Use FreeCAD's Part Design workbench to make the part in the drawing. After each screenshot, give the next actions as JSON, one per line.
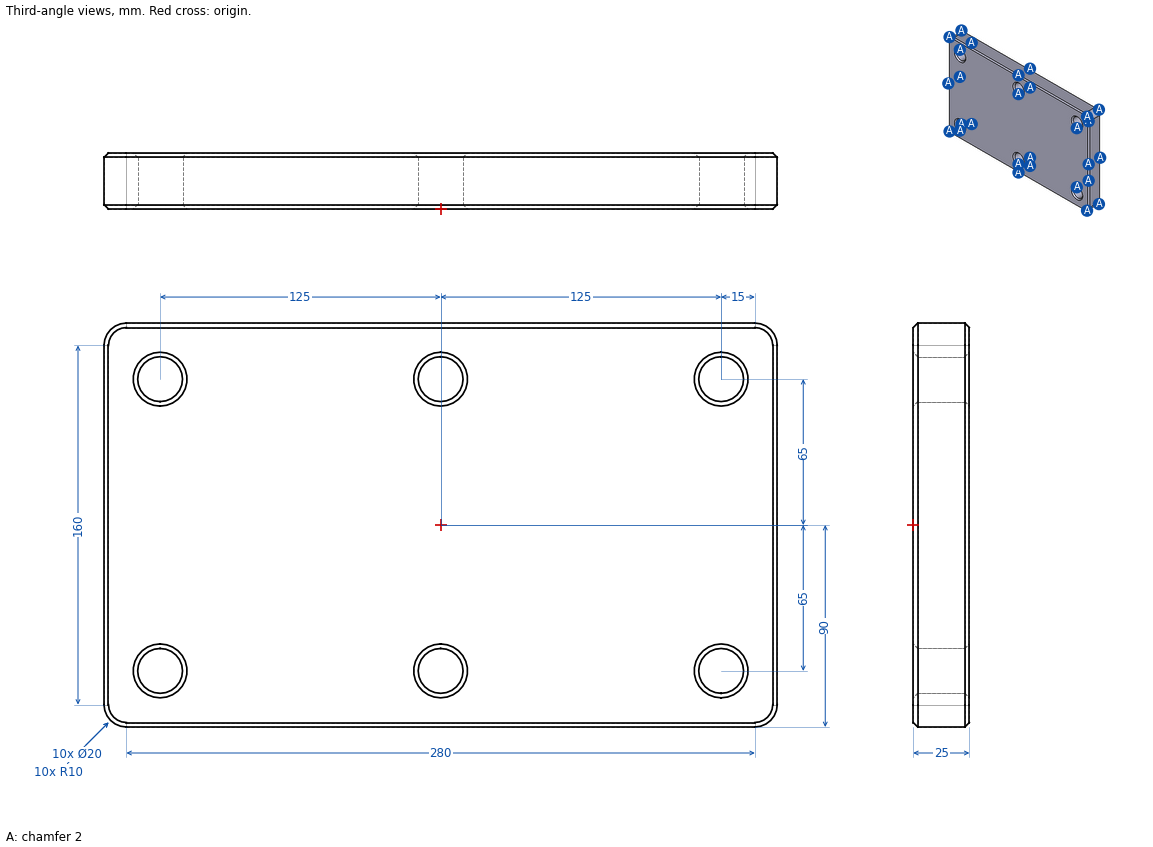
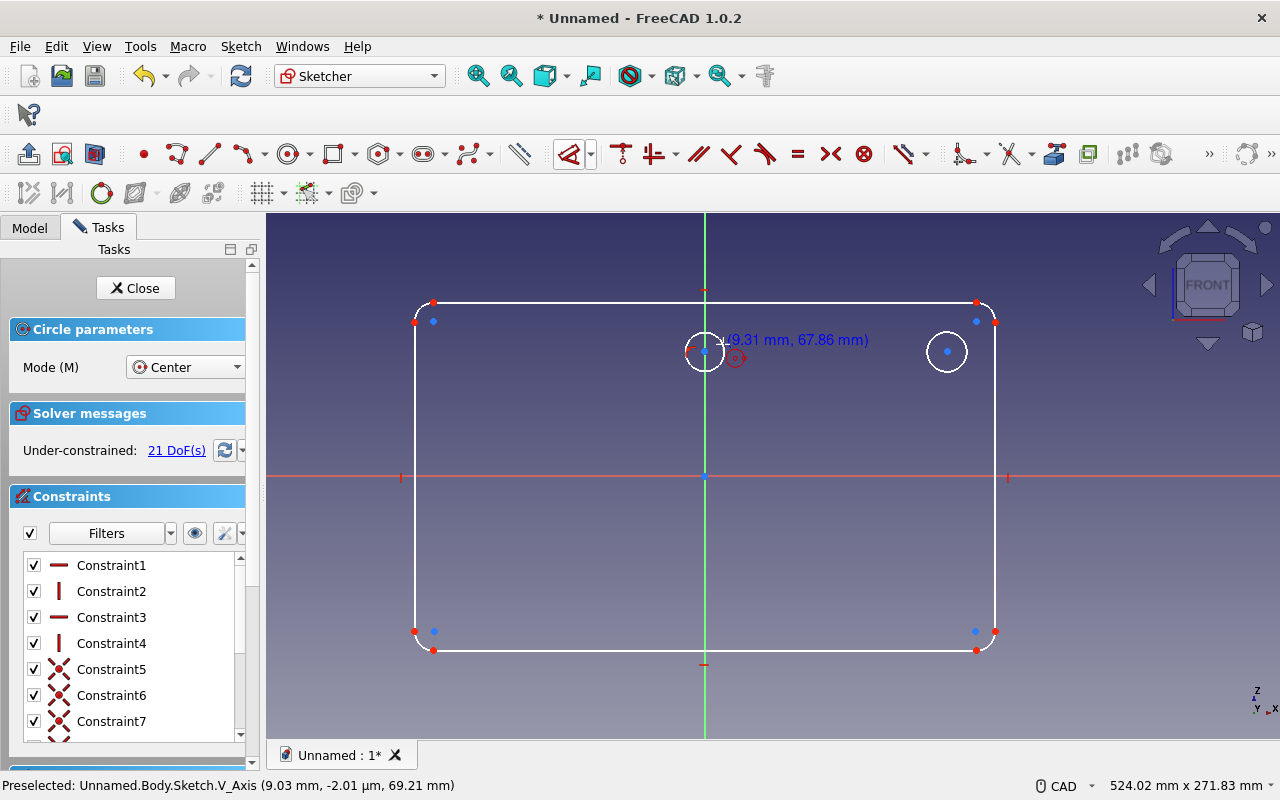
{"action": "left_click", "coordinate": [463, 351]}
{"action": "left_click", "coordinate": [477, 337]}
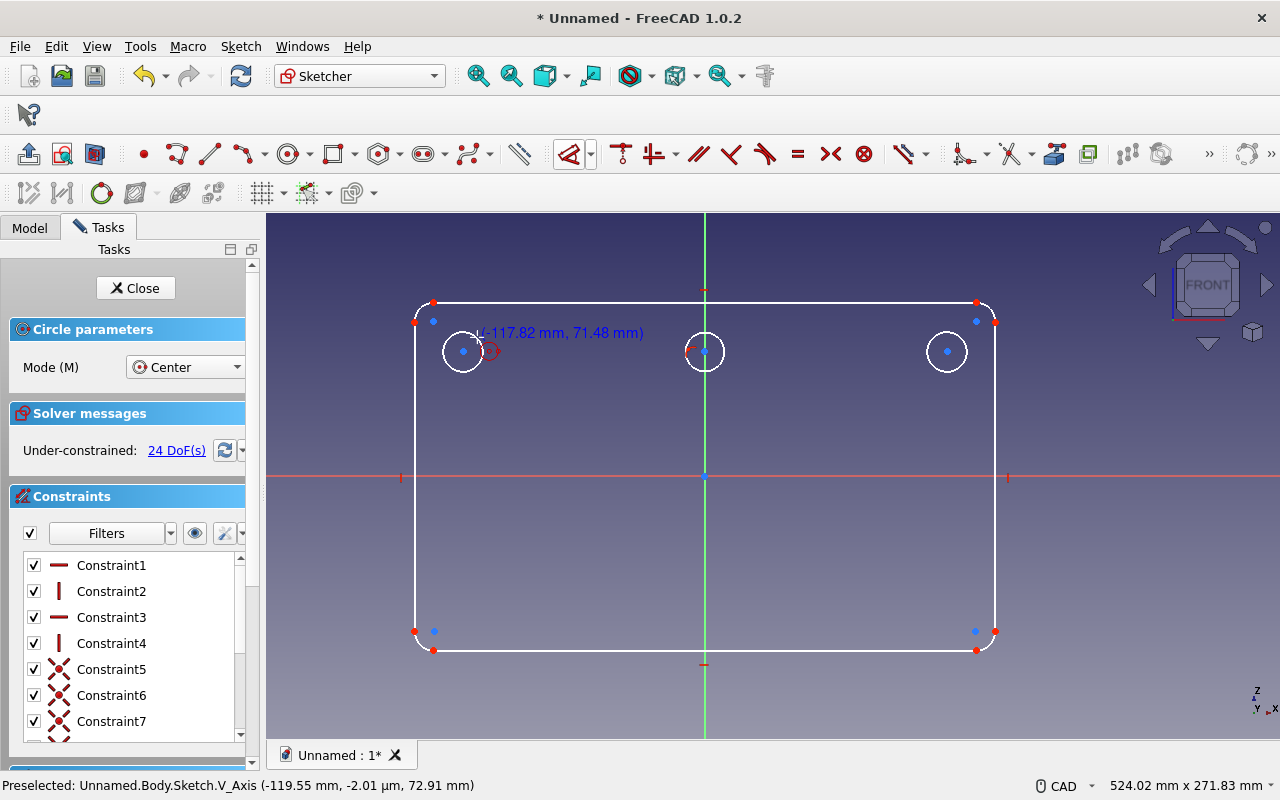
{"action": "left_click", "coordinate": [947, 602]}
{"action": "left_click", "coordinate": [961, 588]}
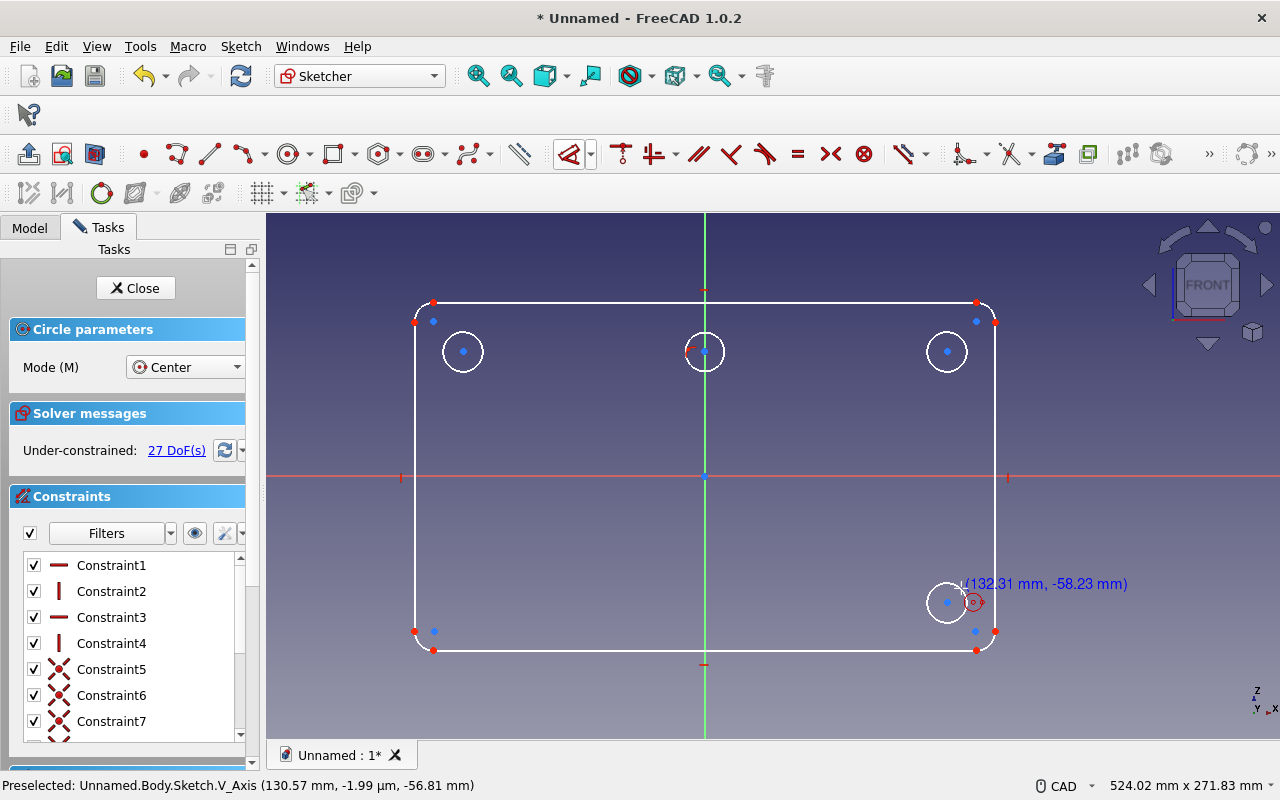
{"action": "left_click", "coordinate": [705, 602]}
{"action": "left_click", "coordinate": [723, 595]}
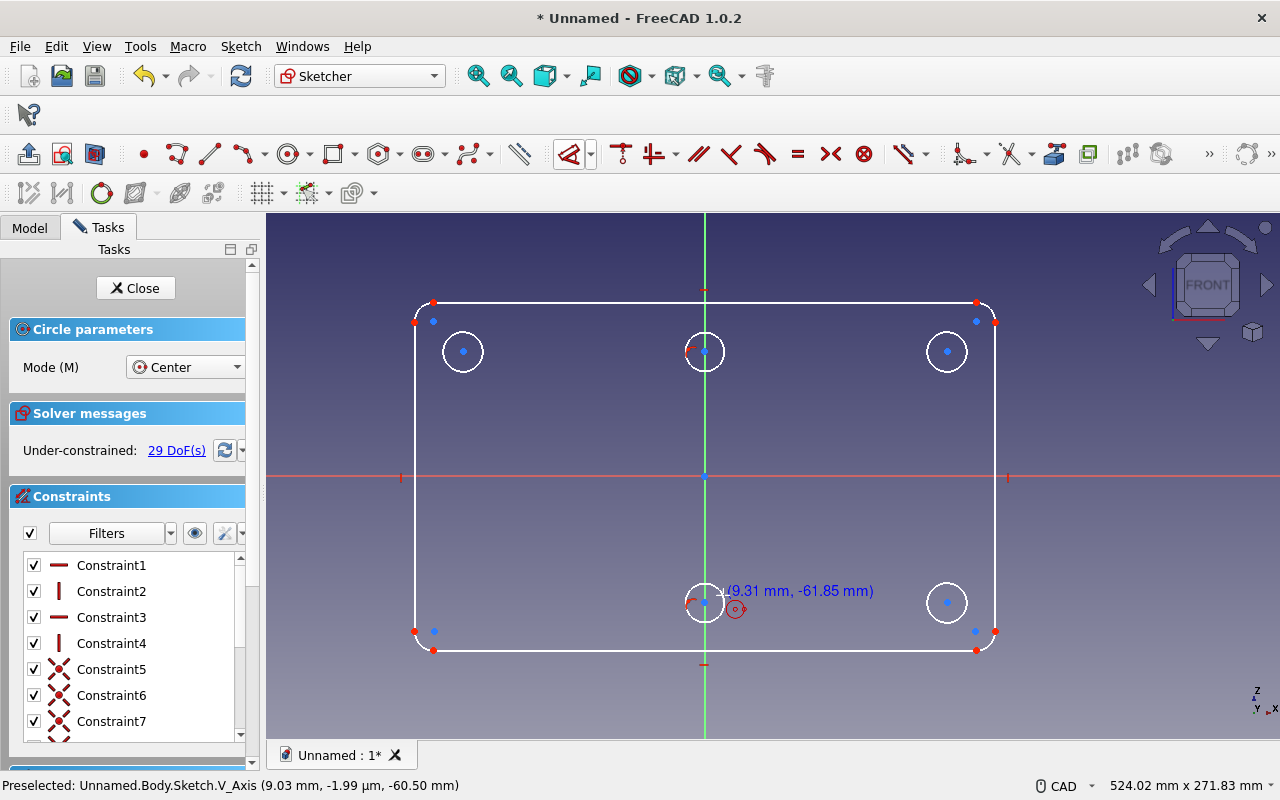
{"action": "left_click", "coordinate": [463, 602]}
{"action": "left_click", "coordinate": [477, 588]}
{"action": "key", "text": "Escape"}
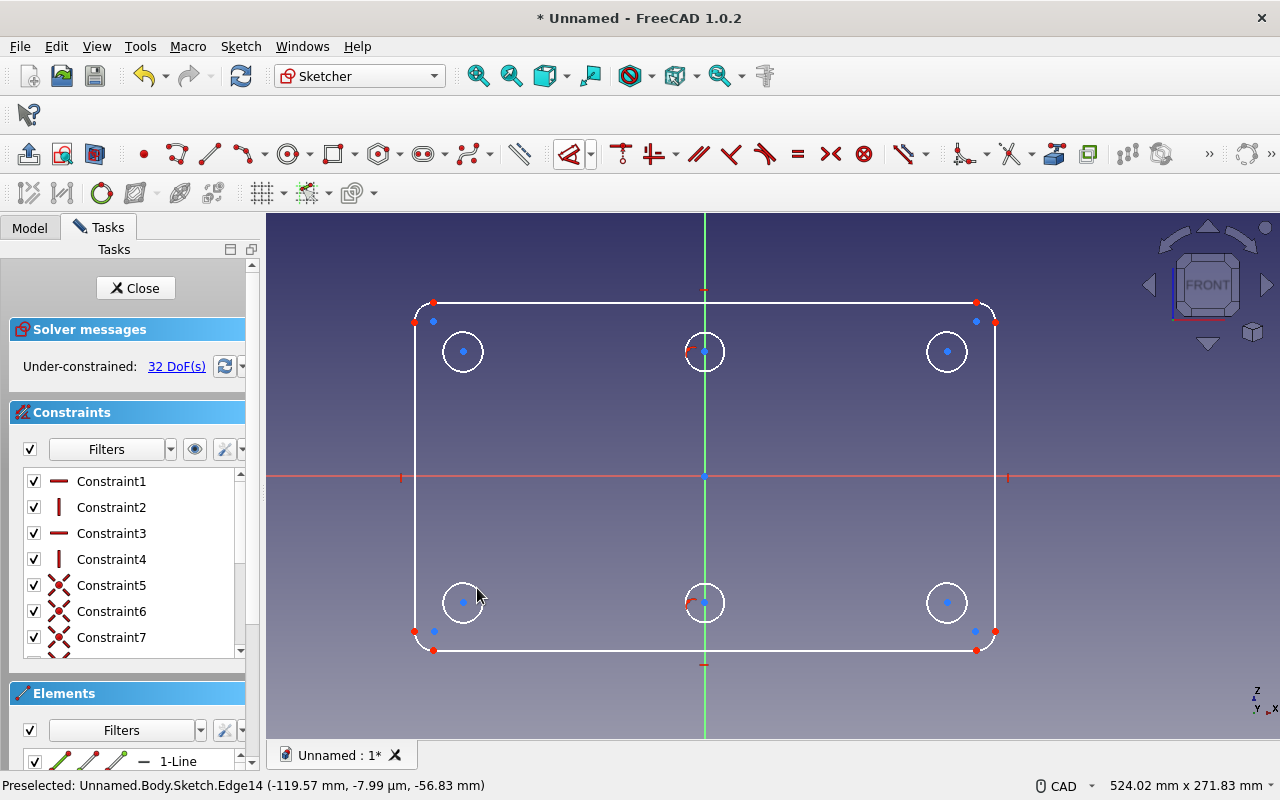
{"action": "left_click", "coordinate": [813, 651]}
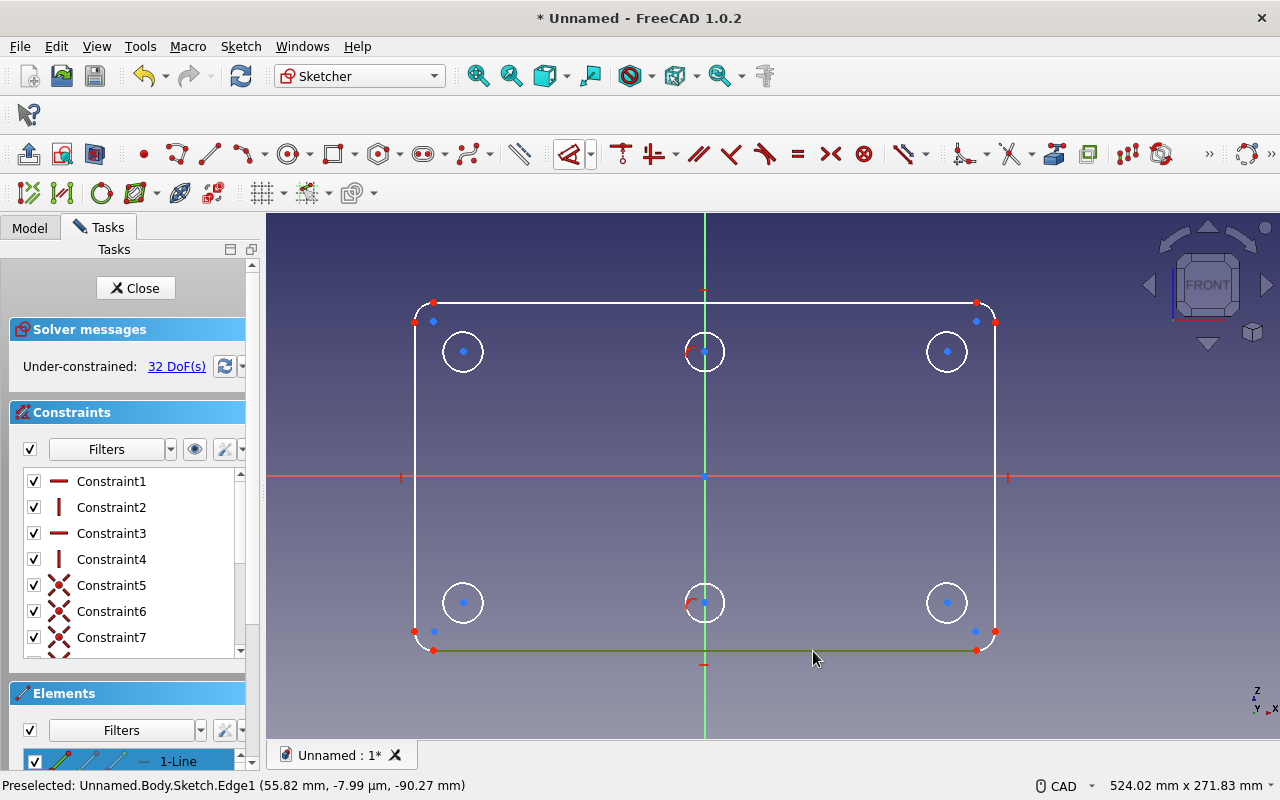
{"action": "left_click", "coordinate": [421, 645]}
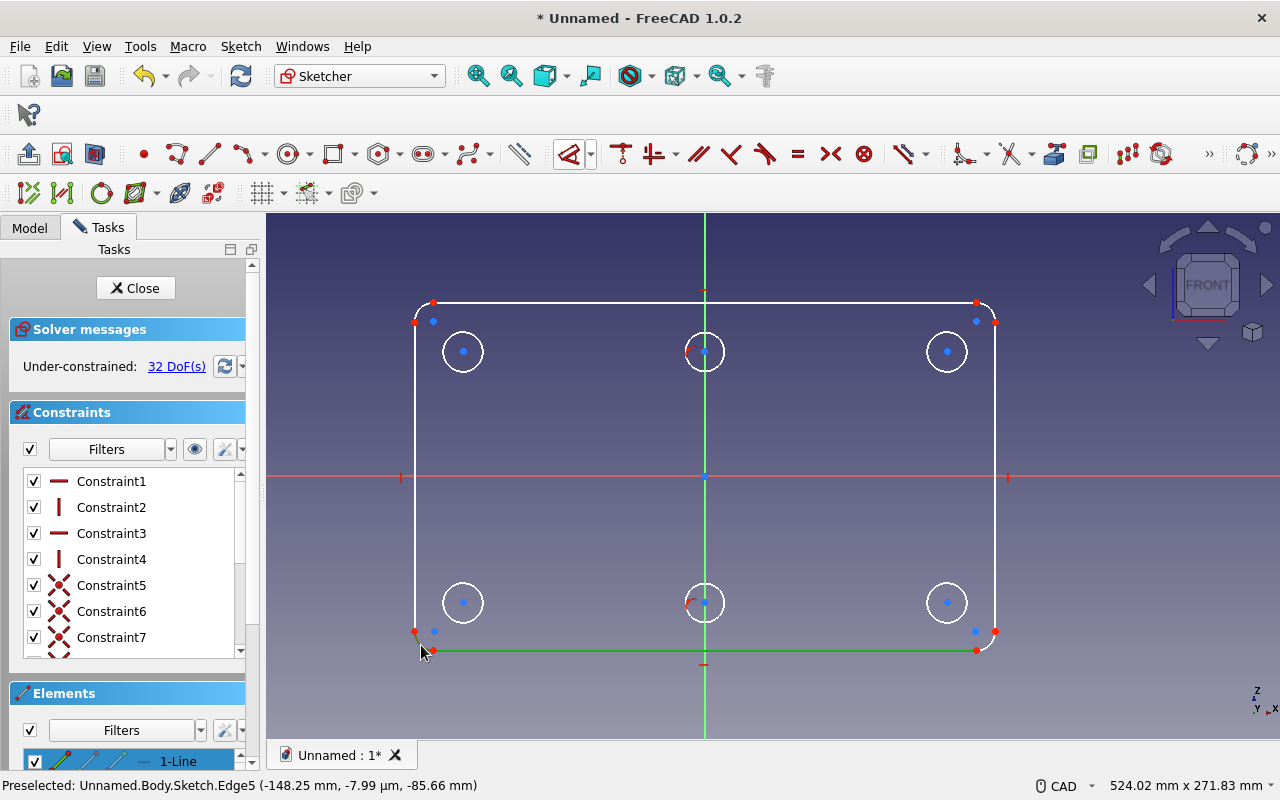
{"action": "left_click", "coordinate": [765, 154]}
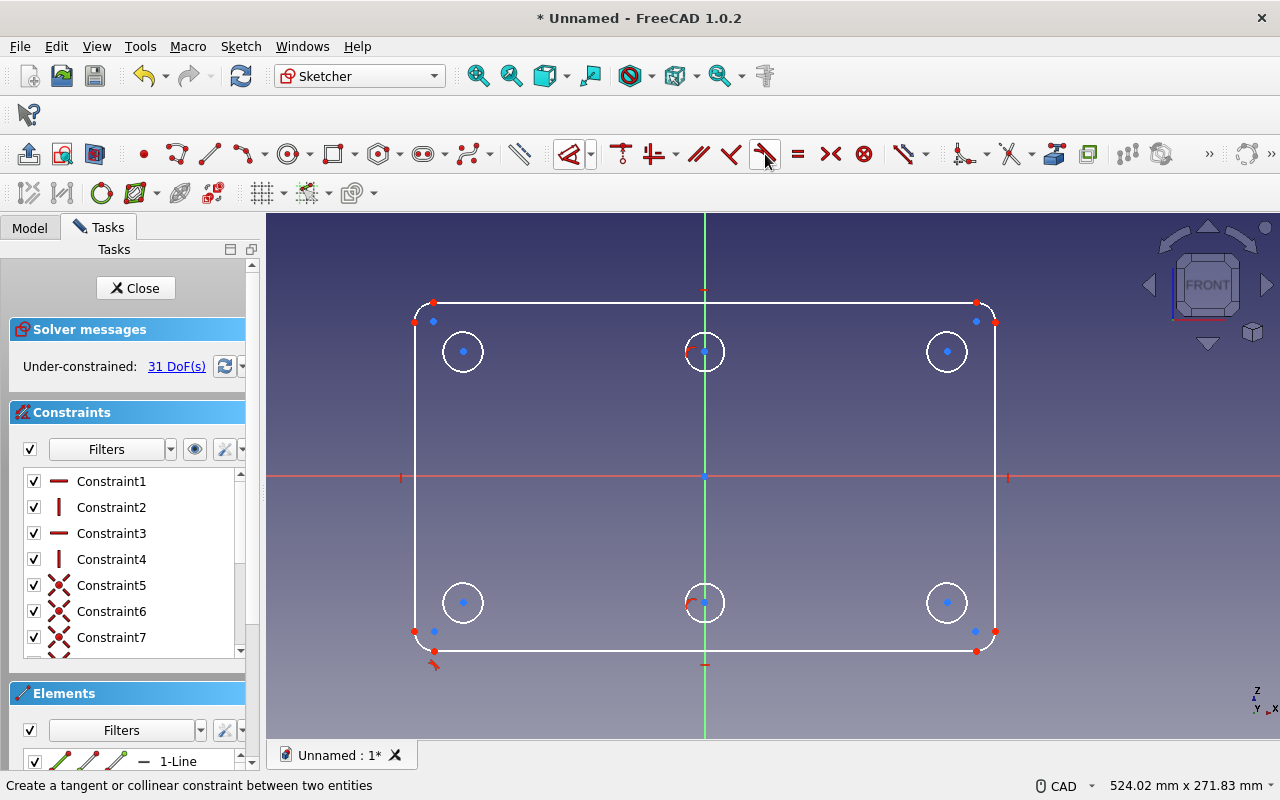
{"action": "left_click", "coordinate": [814, 651]}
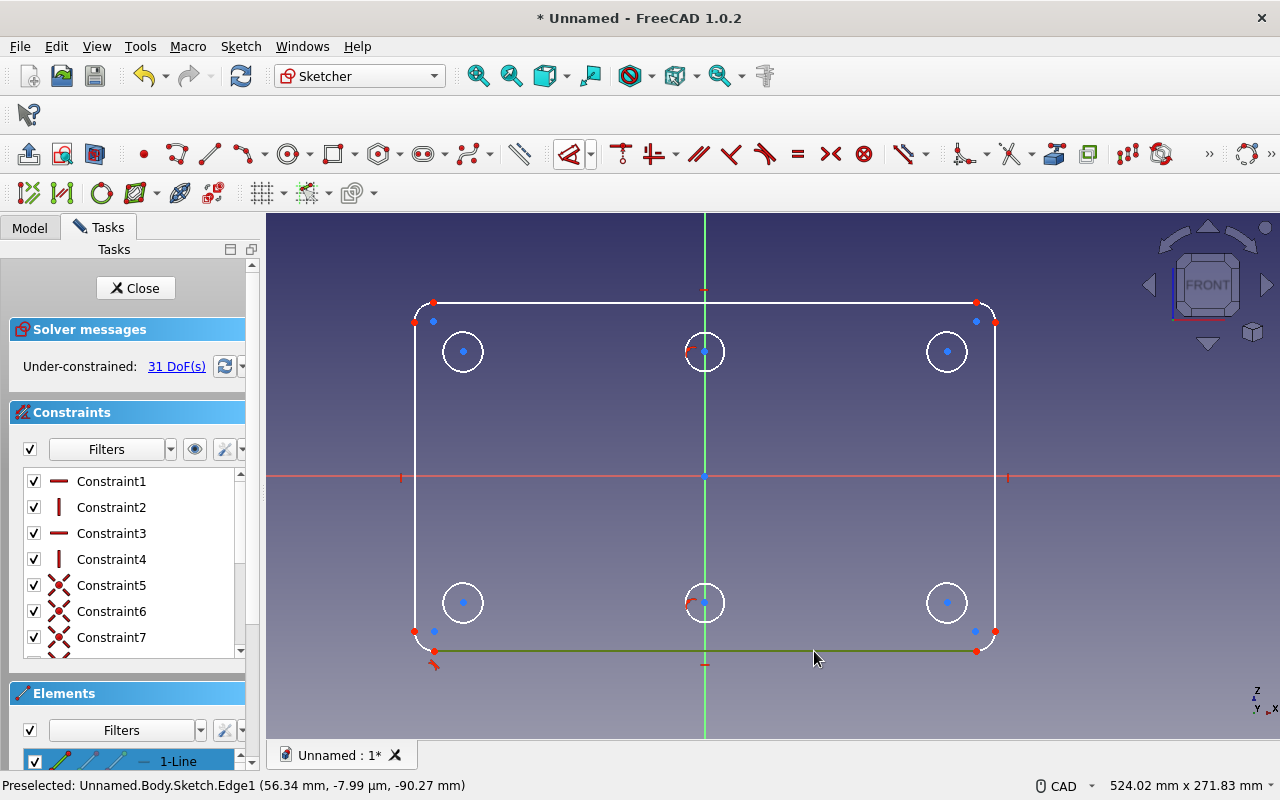
{"action": "left_click", "coordinate": [989, 645]}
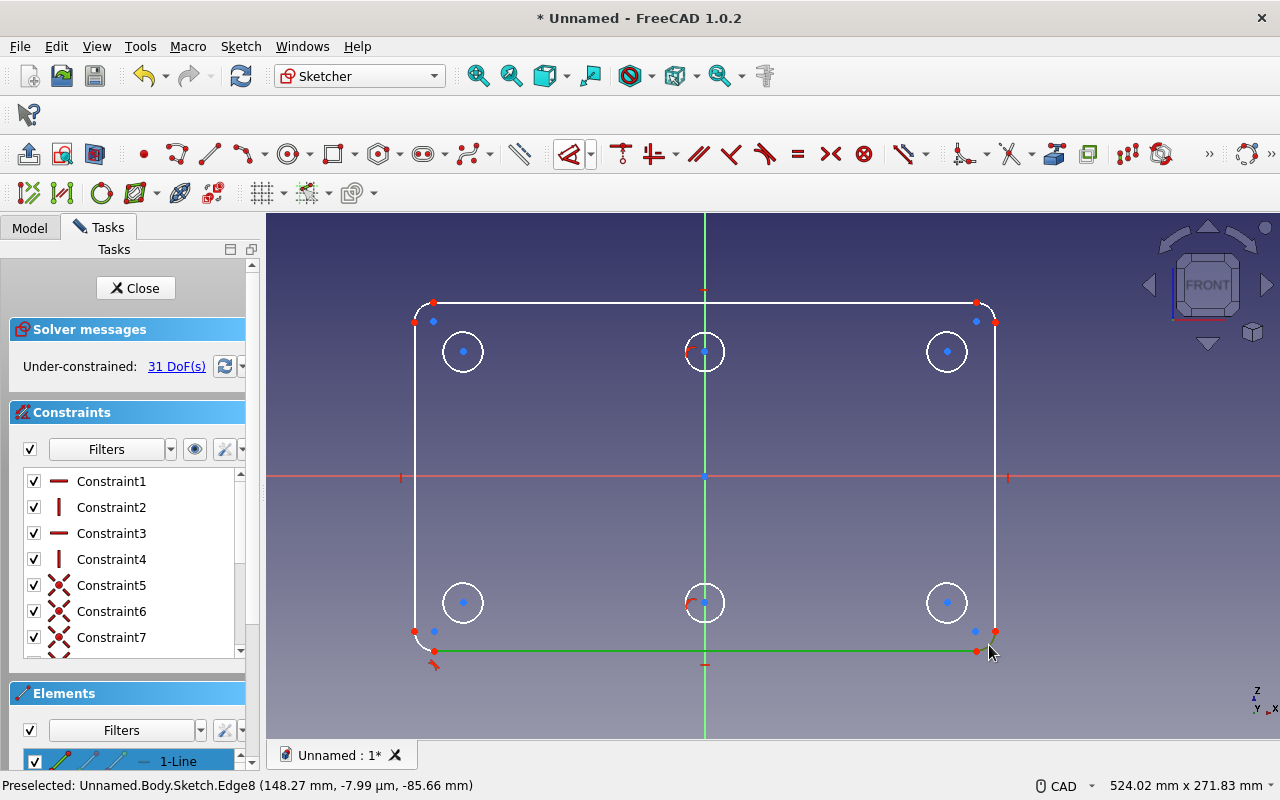
{"action": "left_click", "coordinate": [765, 154]}